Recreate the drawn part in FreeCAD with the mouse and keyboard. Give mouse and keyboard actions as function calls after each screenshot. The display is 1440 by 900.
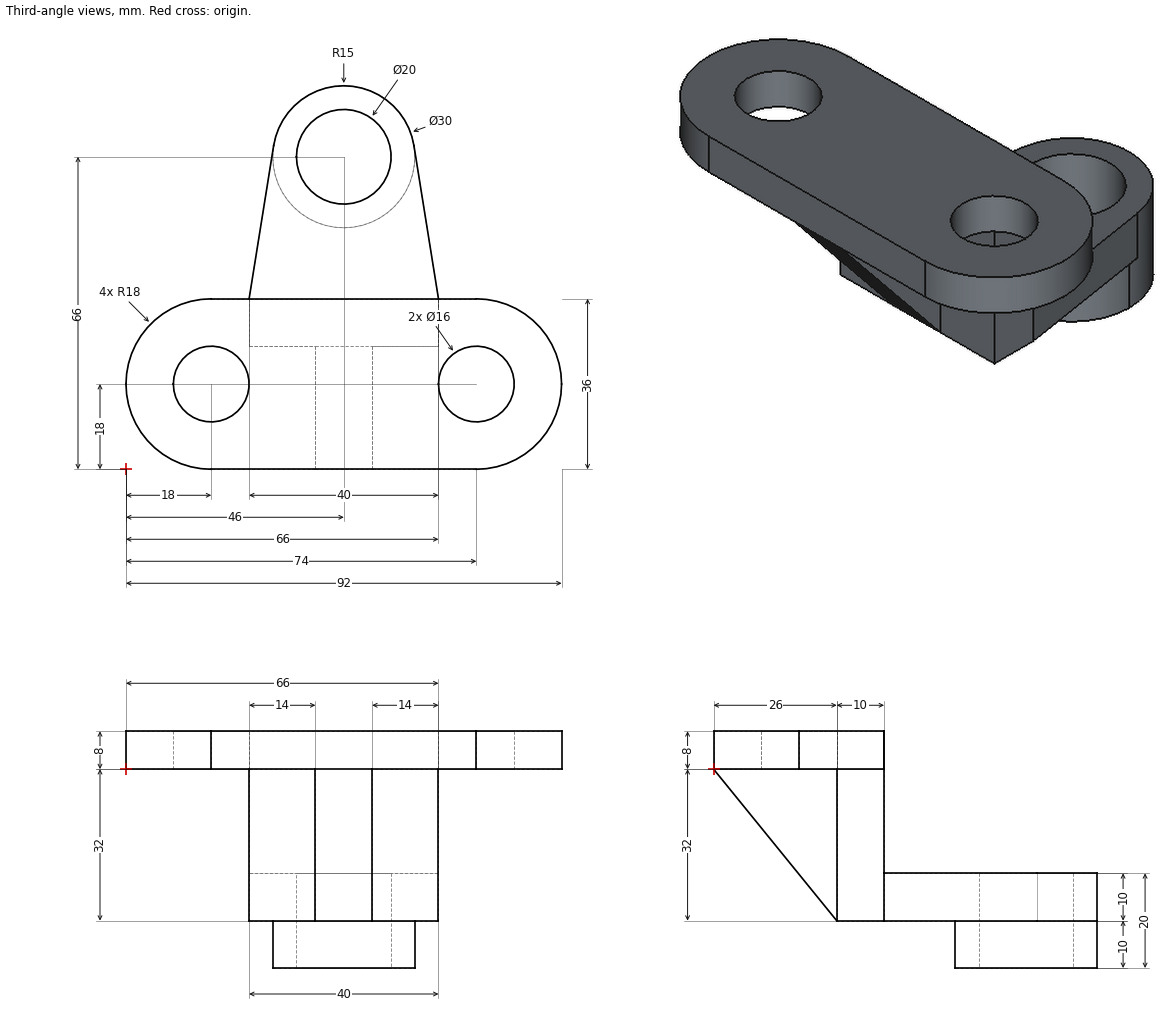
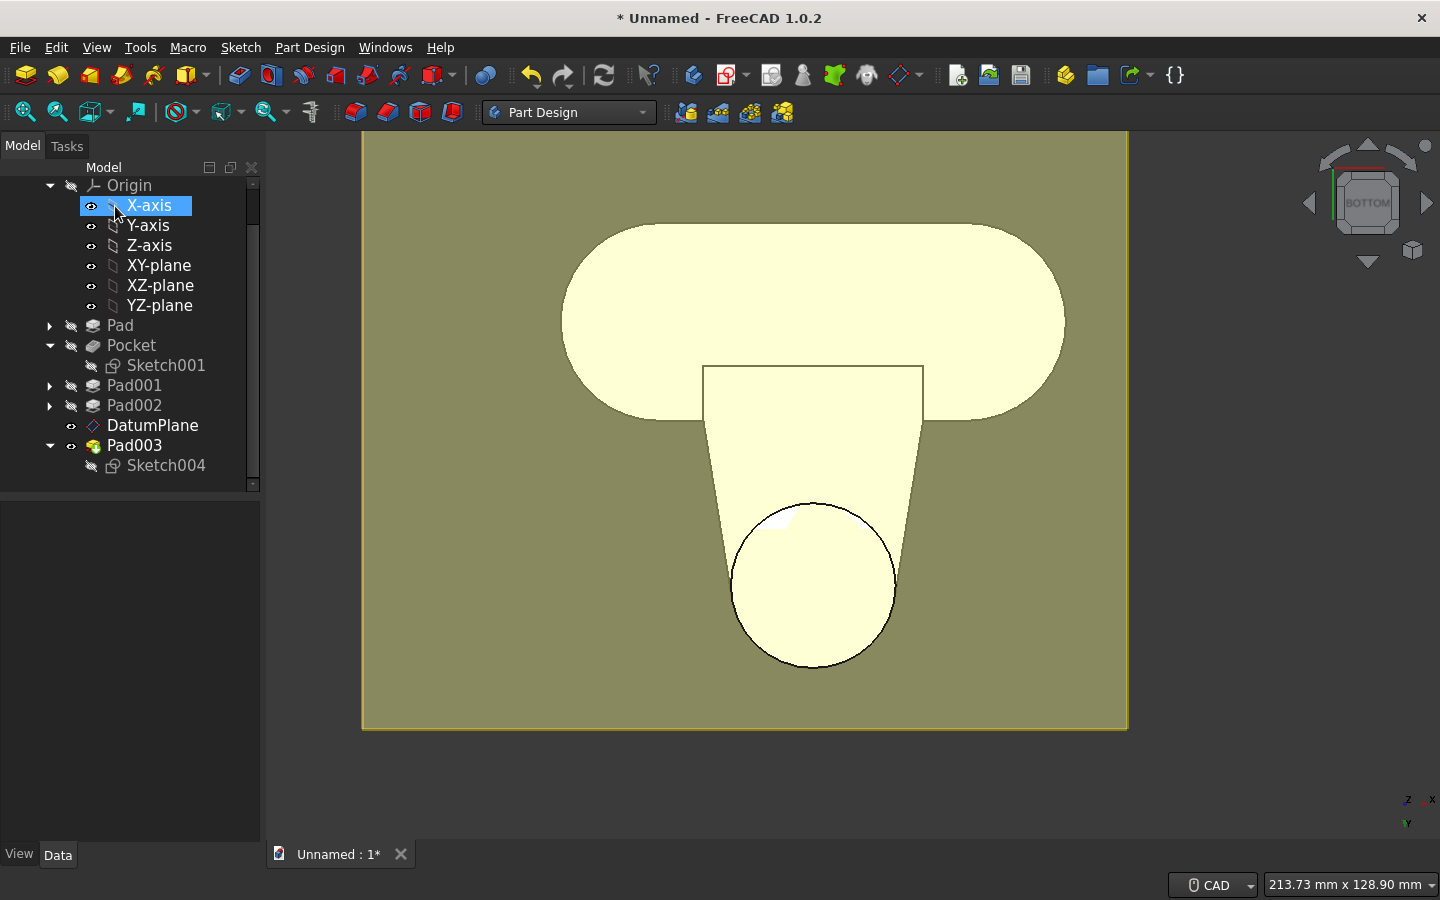
click(116, 426)
key(space)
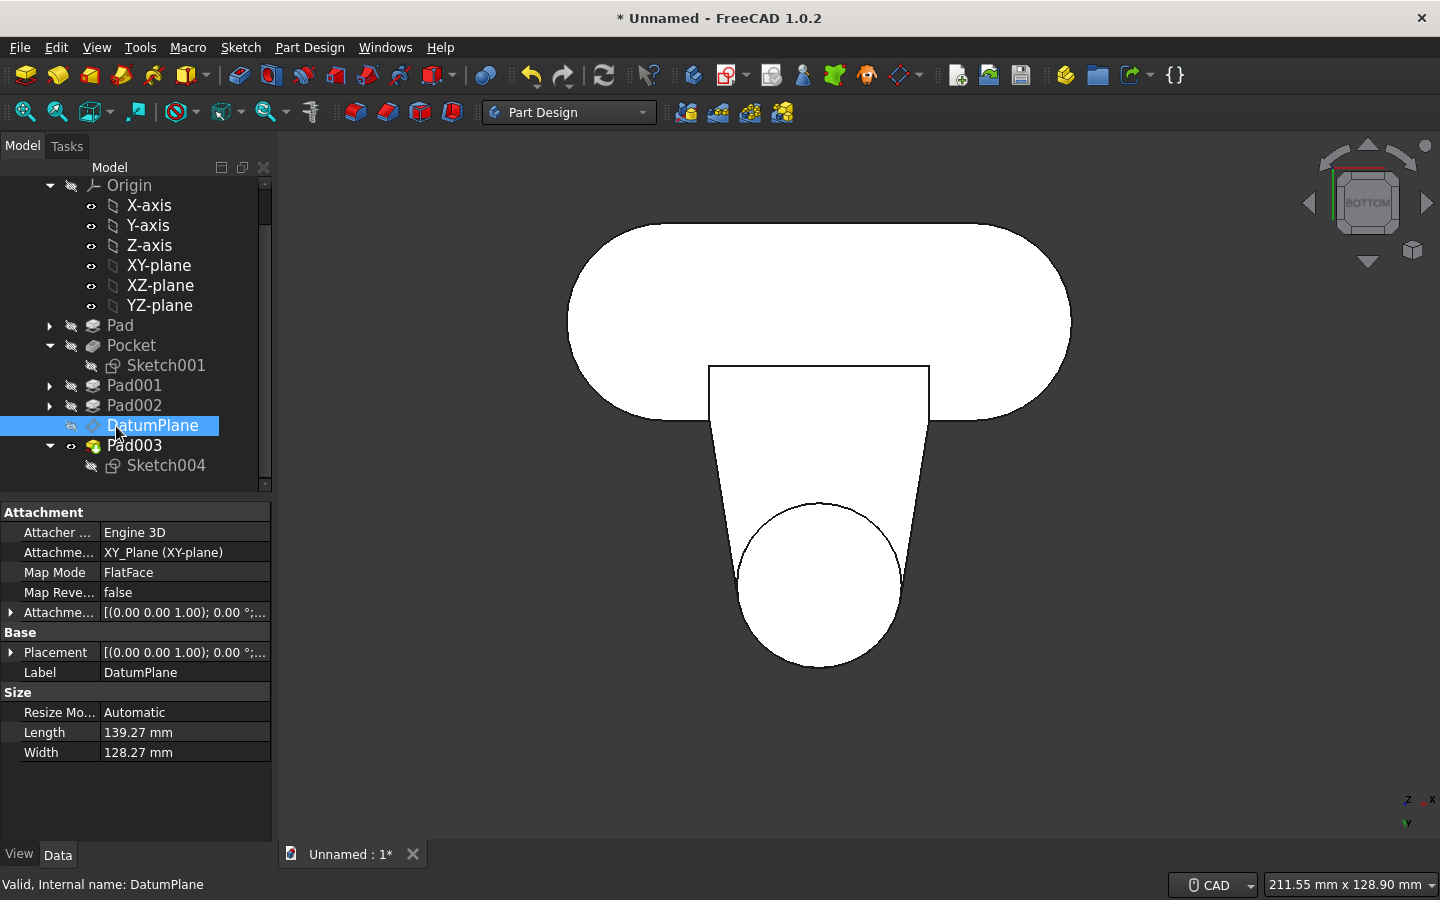
click(819, 585)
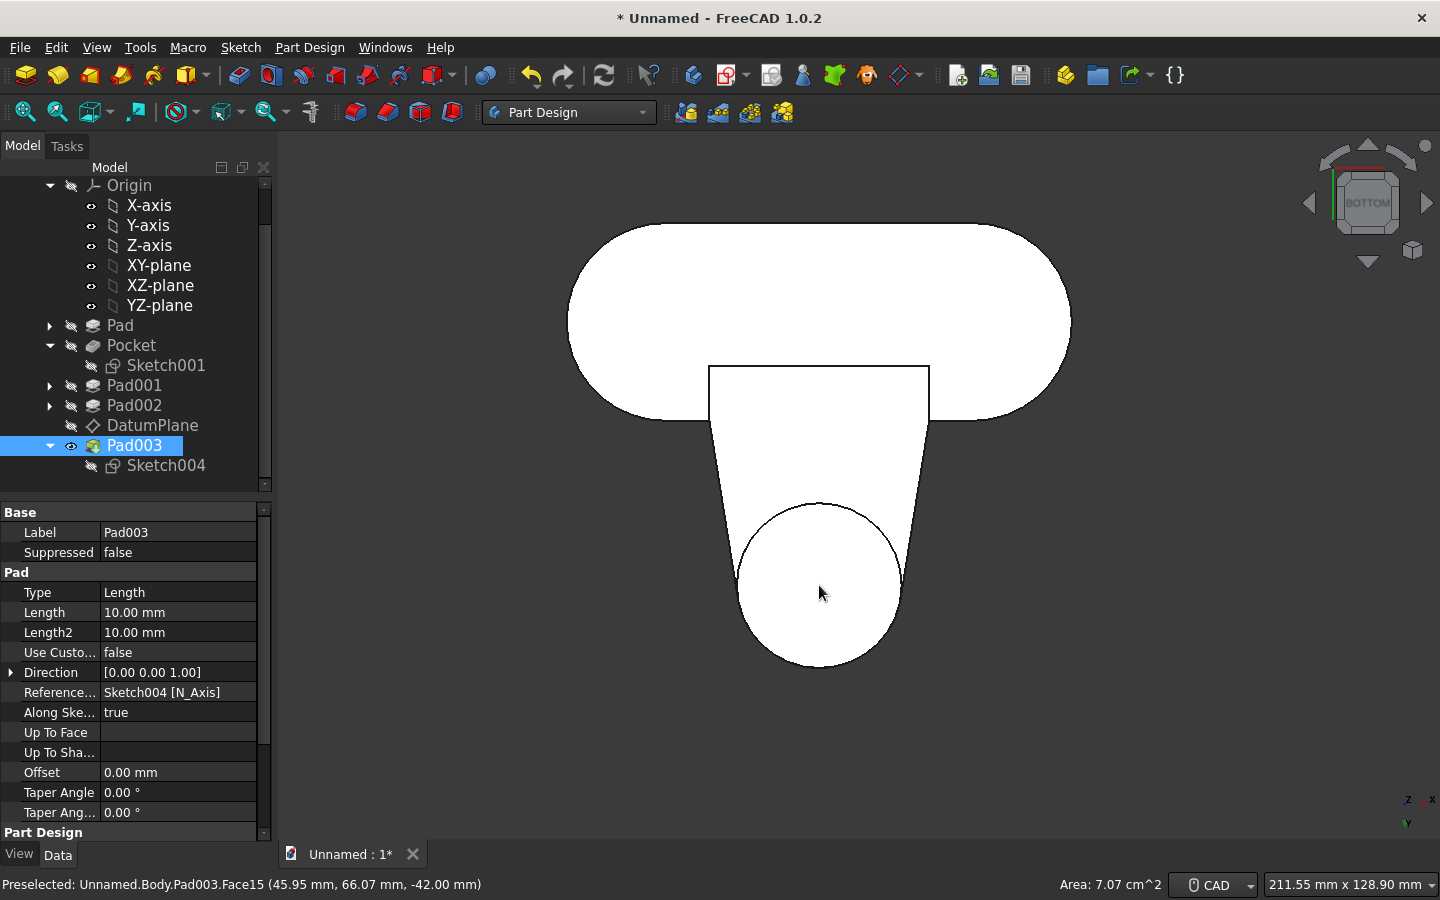
click(726, 76)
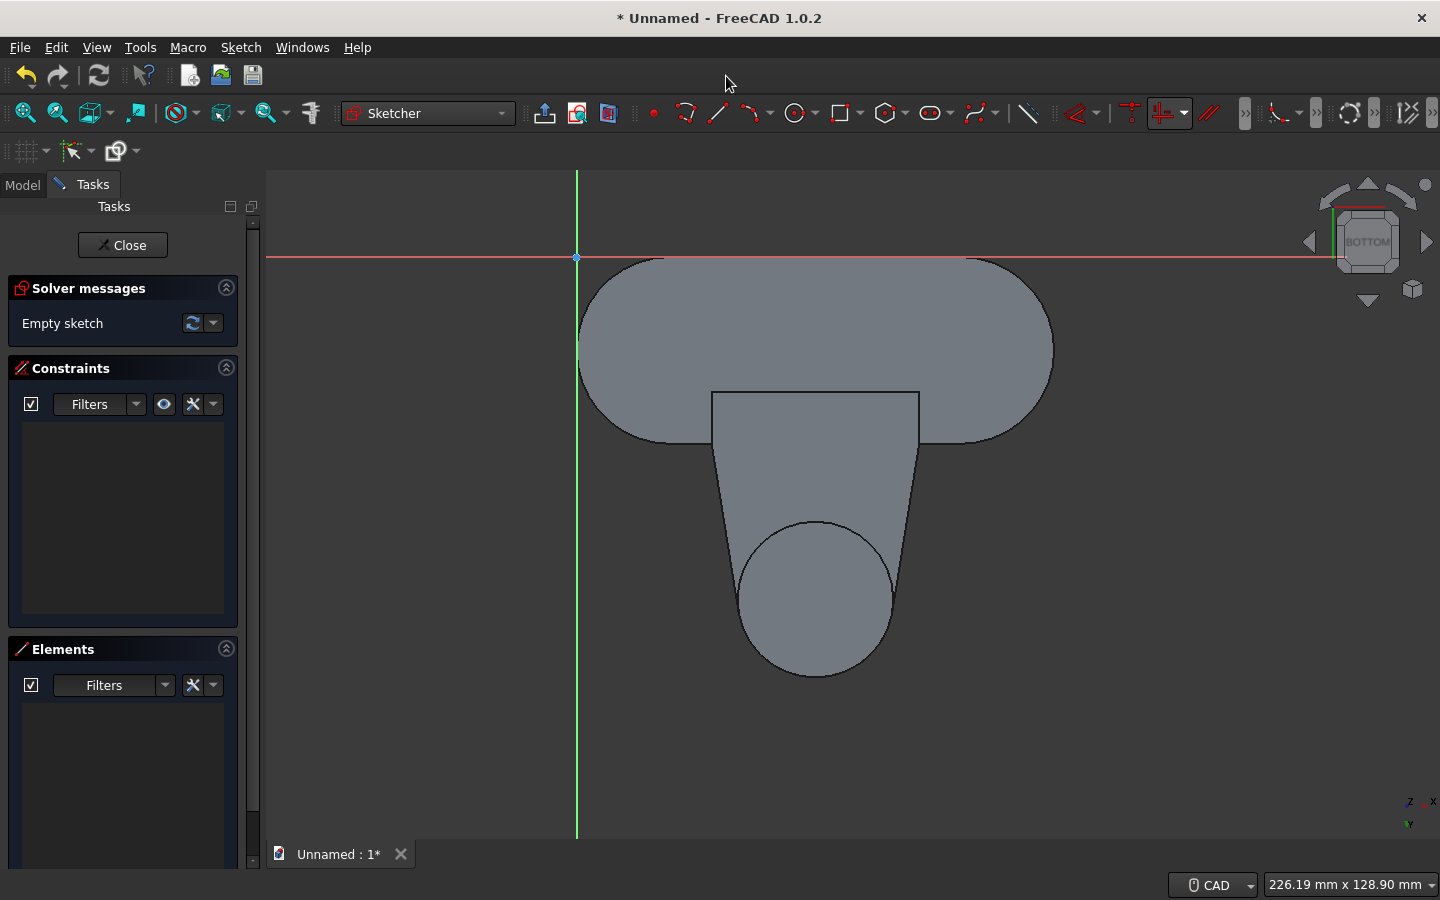
scroll(826, 631, up, 7)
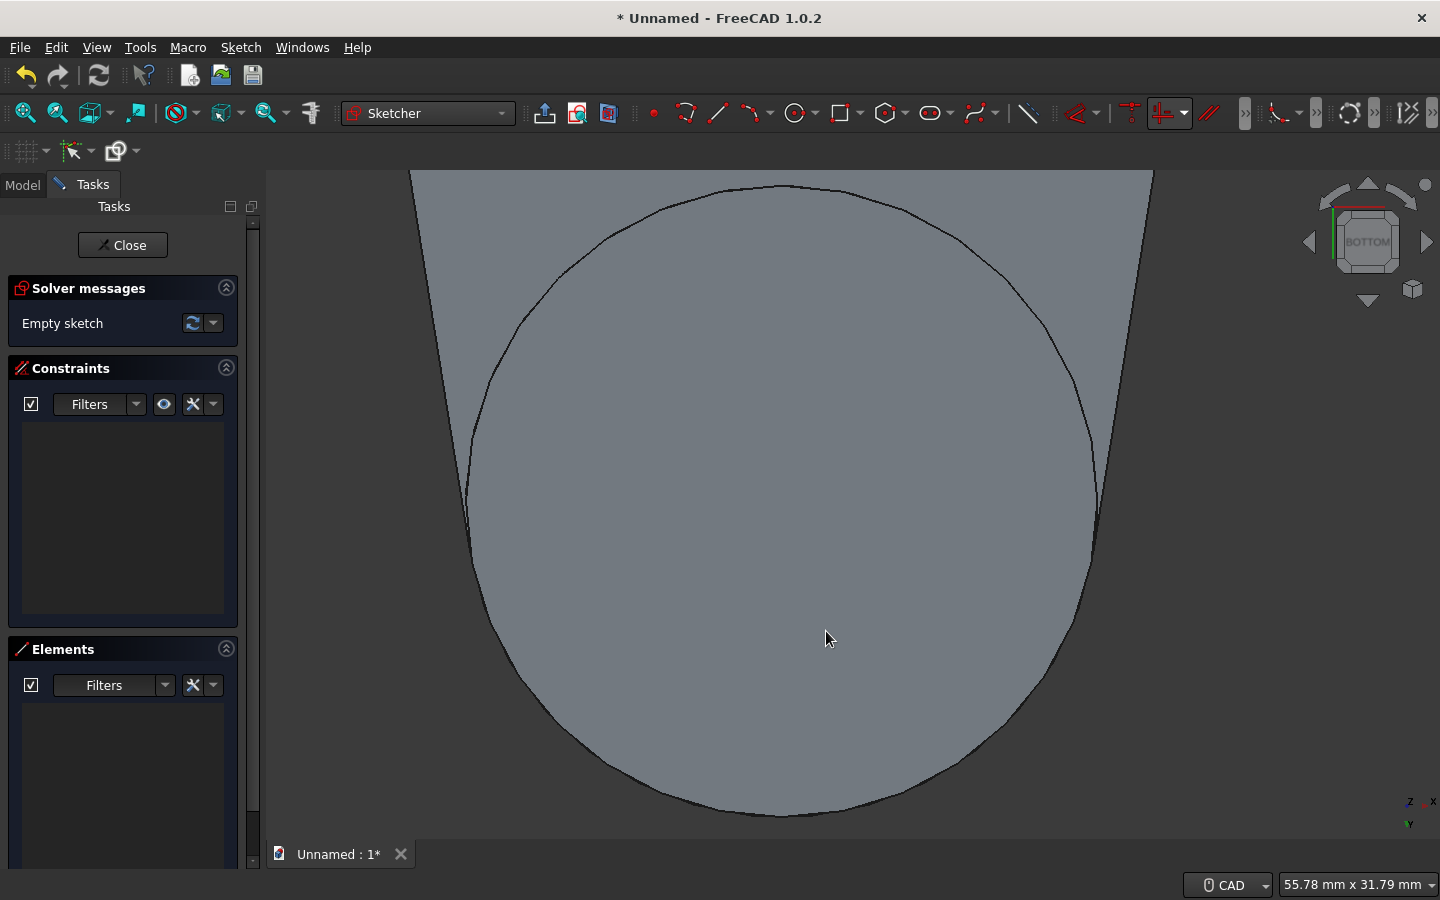
click(796, 114)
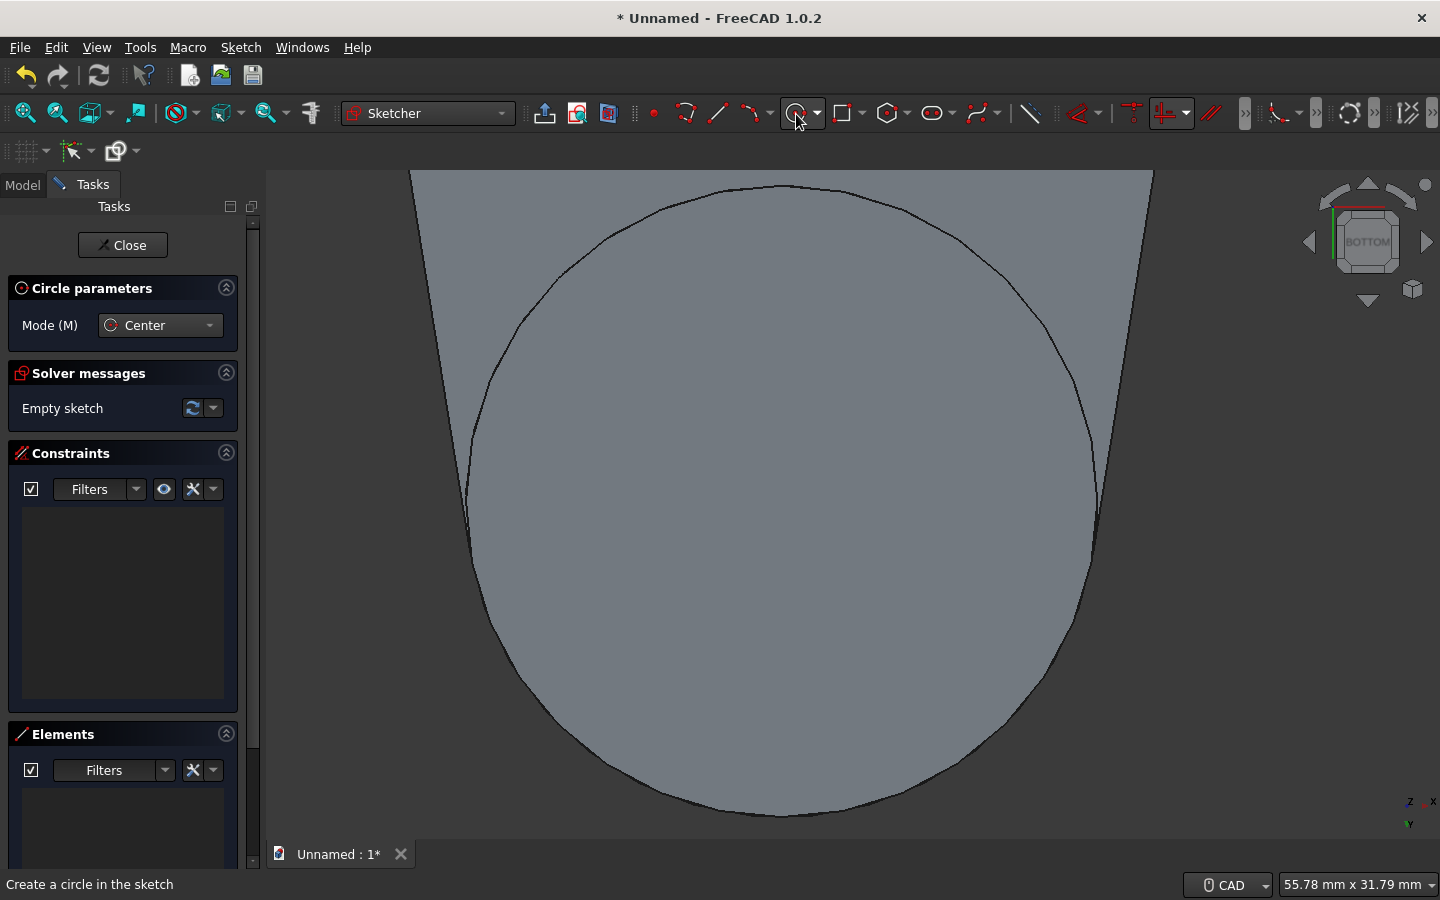
click(782, 501)
move(931, 353)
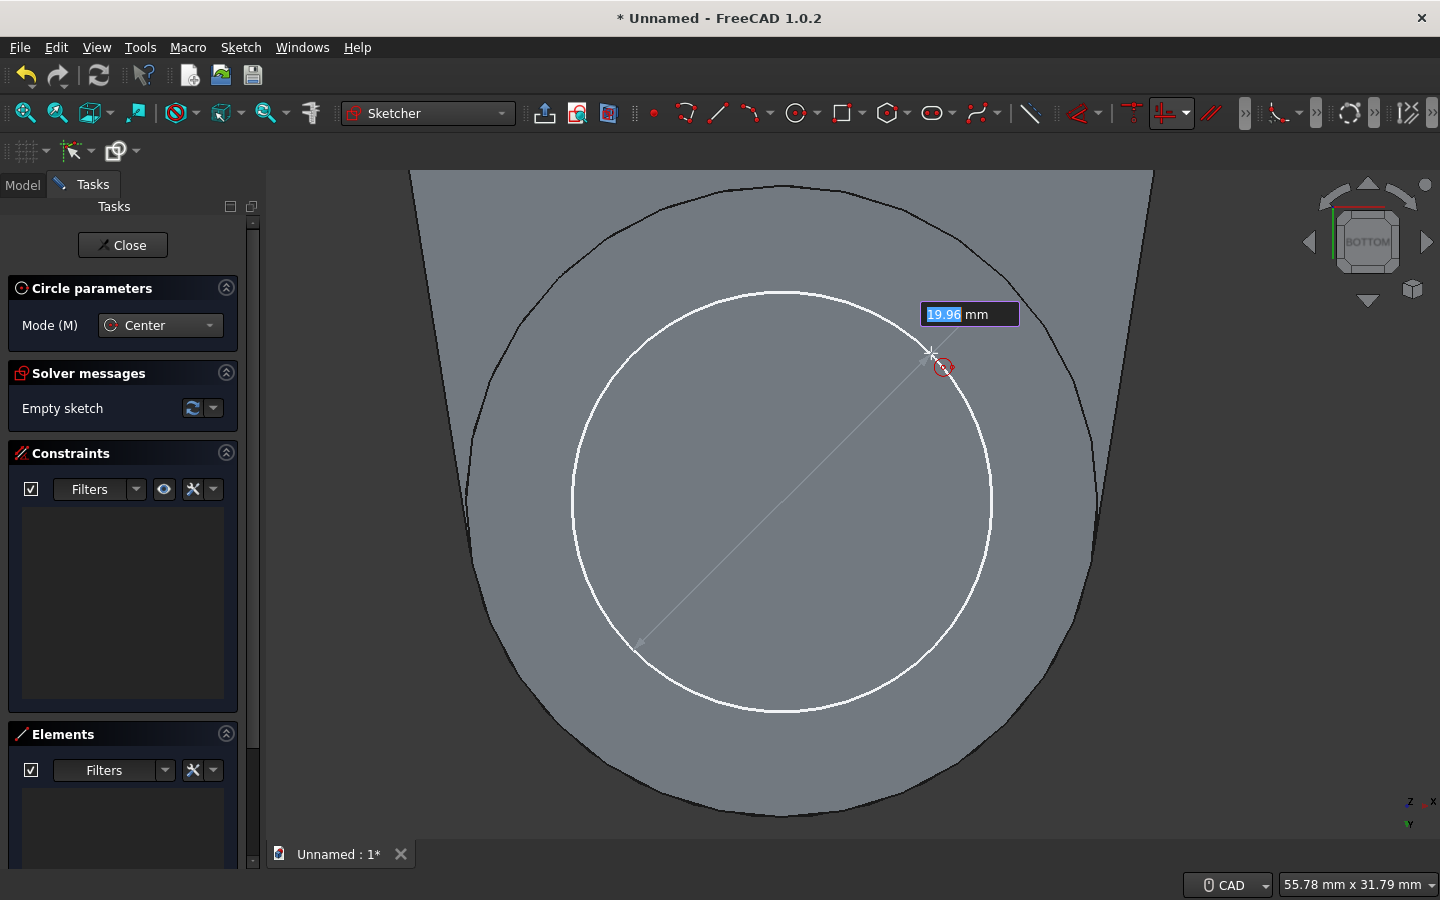
text(20)
key(Return)
key(Escape)